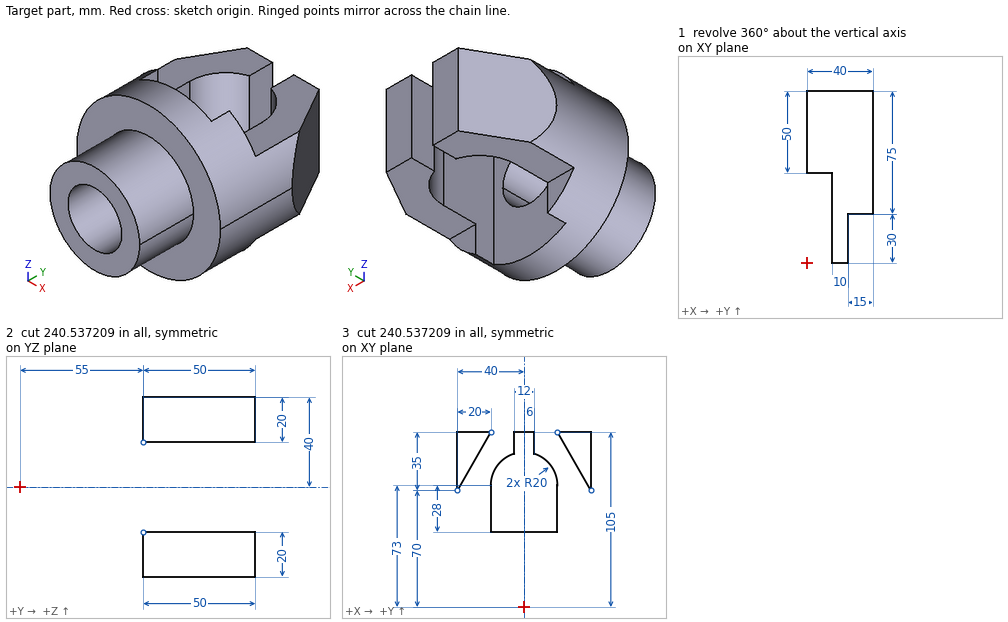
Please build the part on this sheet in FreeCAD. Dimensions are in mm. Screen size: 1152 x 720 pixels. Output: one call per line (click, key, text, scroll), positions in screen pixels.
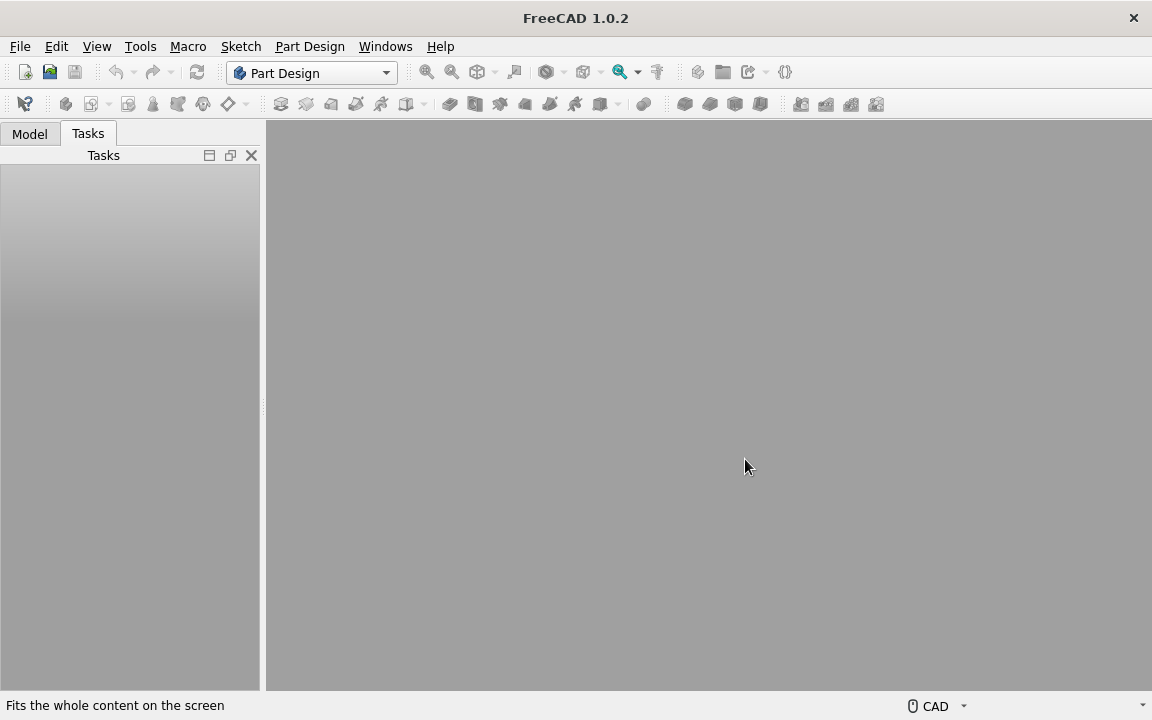
click(25, 72)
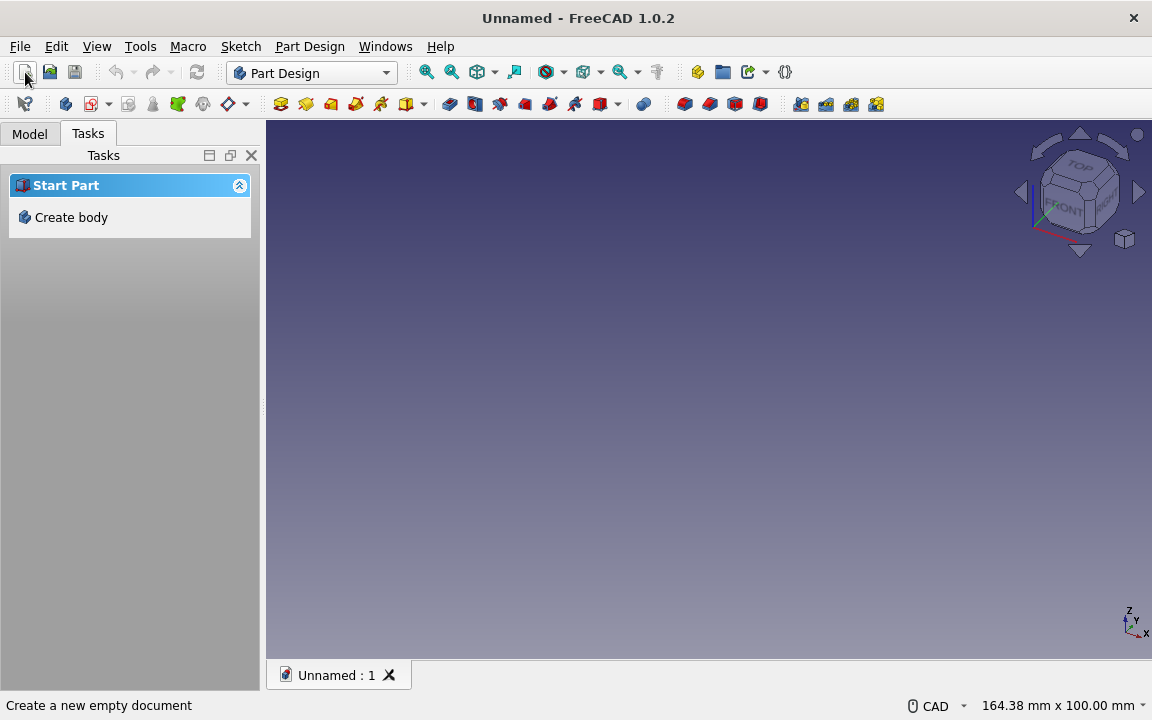
click(90, 104)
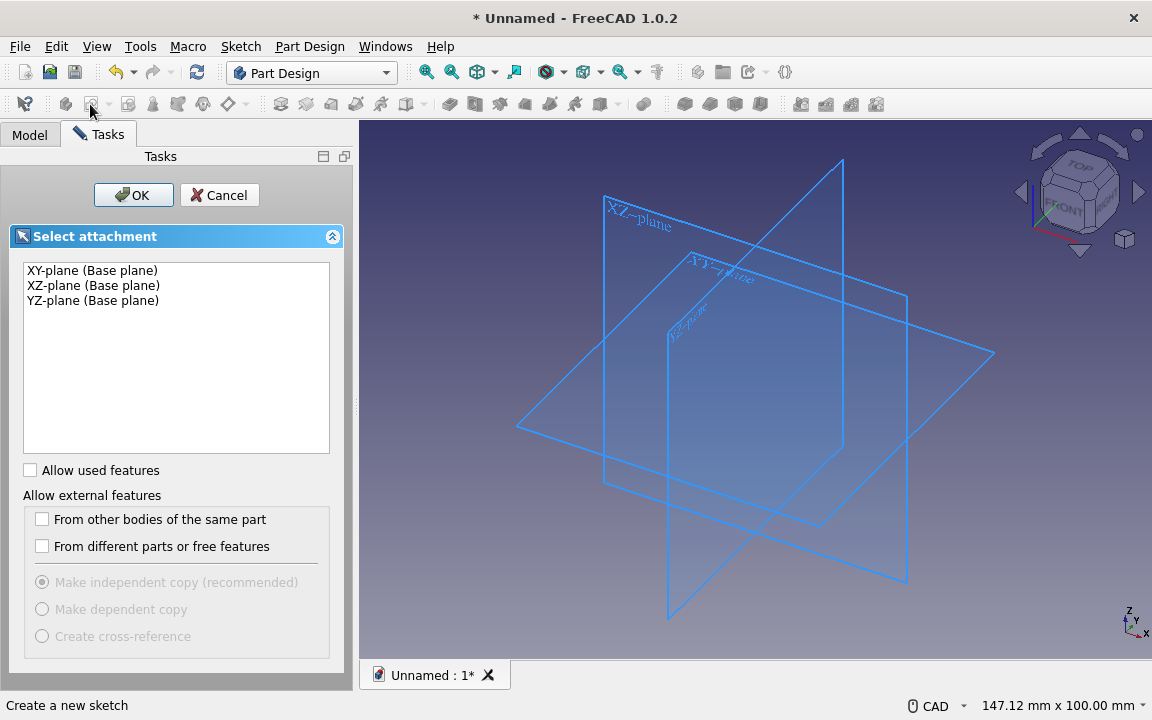
click(84, 270)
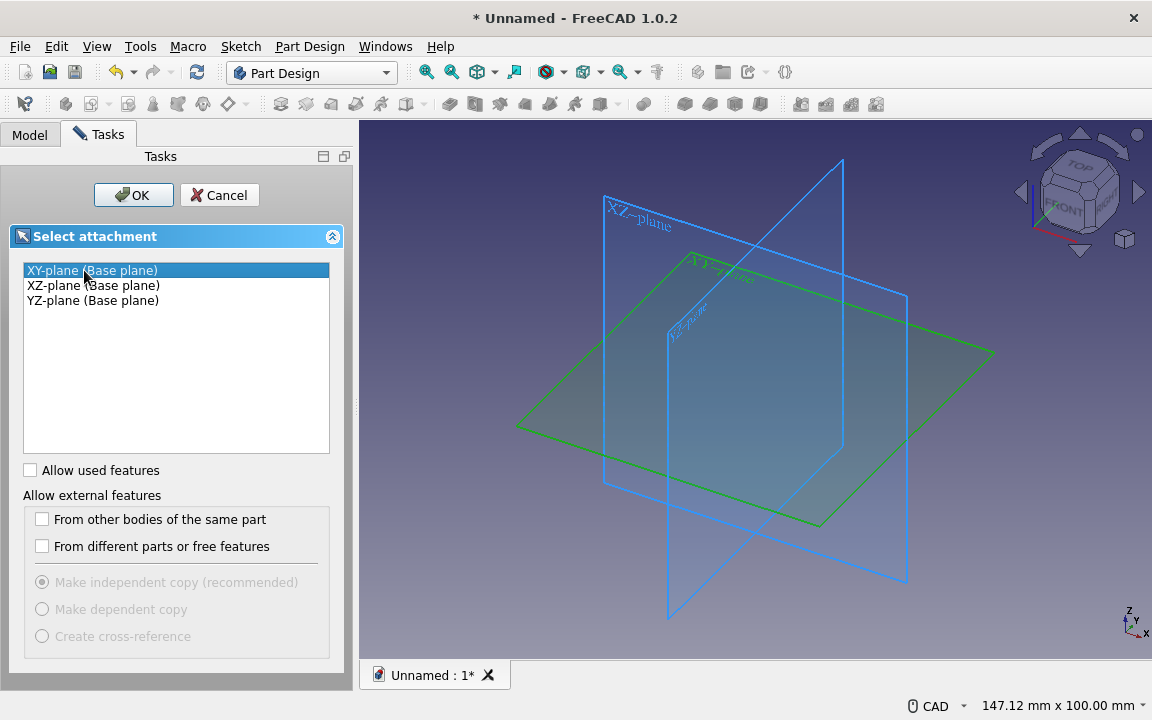
click(134, 195)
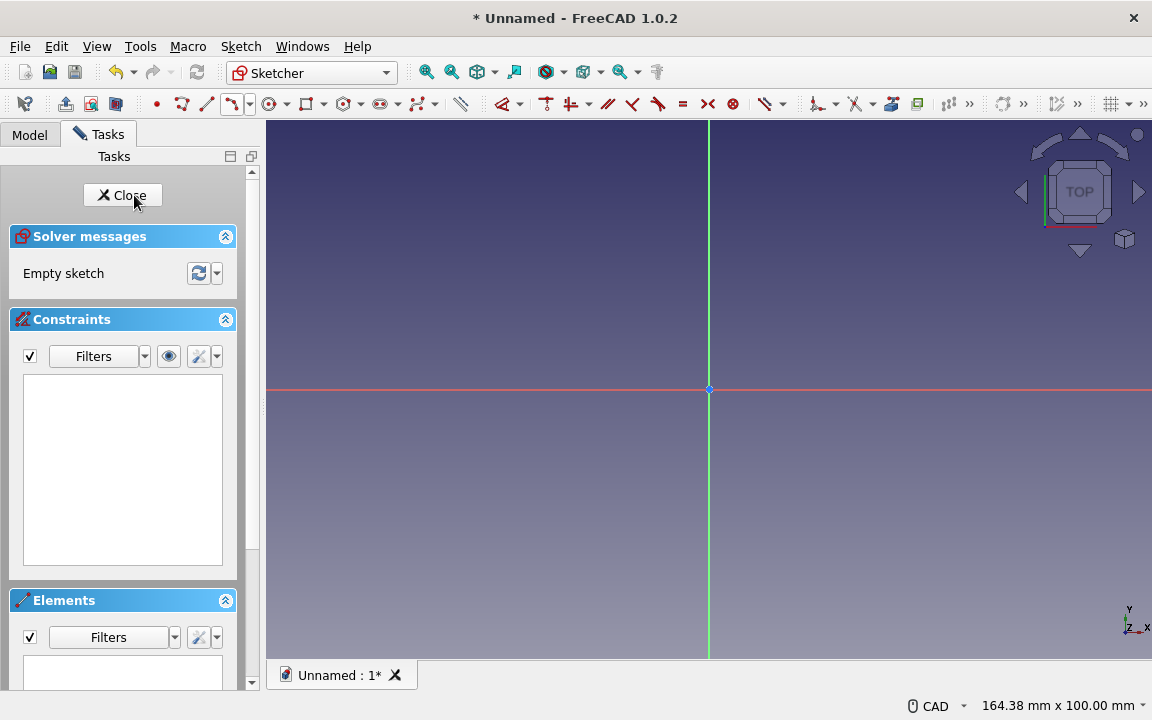
scroll(426, 631, down, 3)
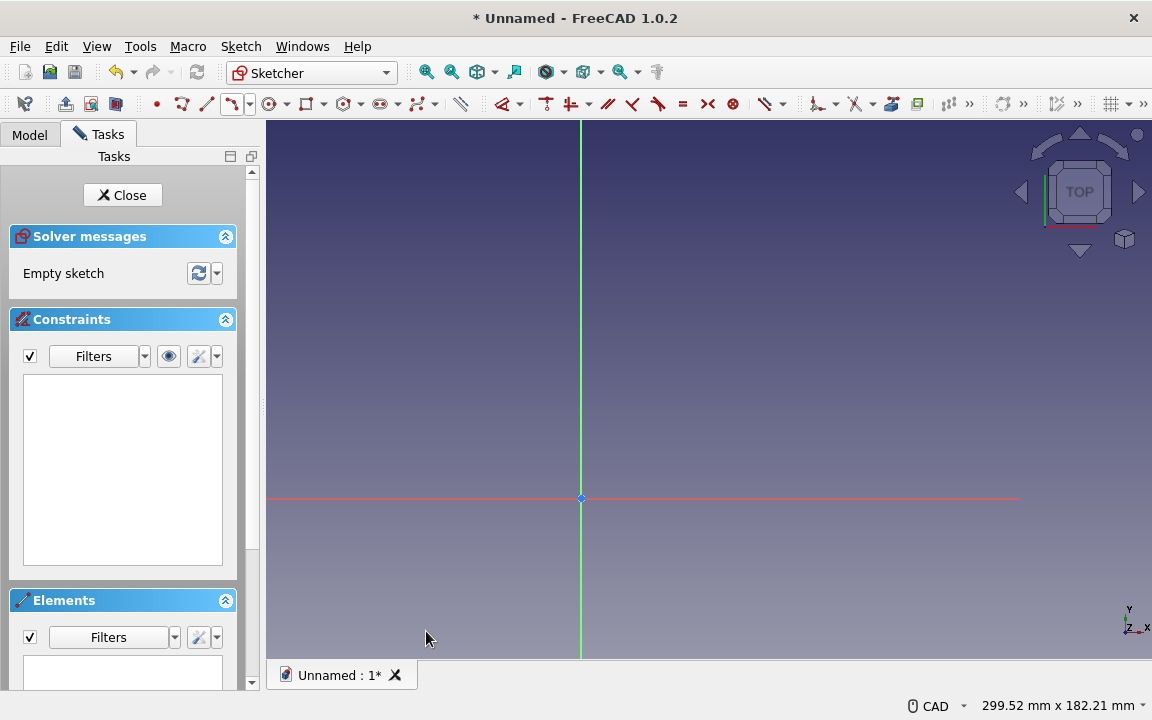
click(182, 104)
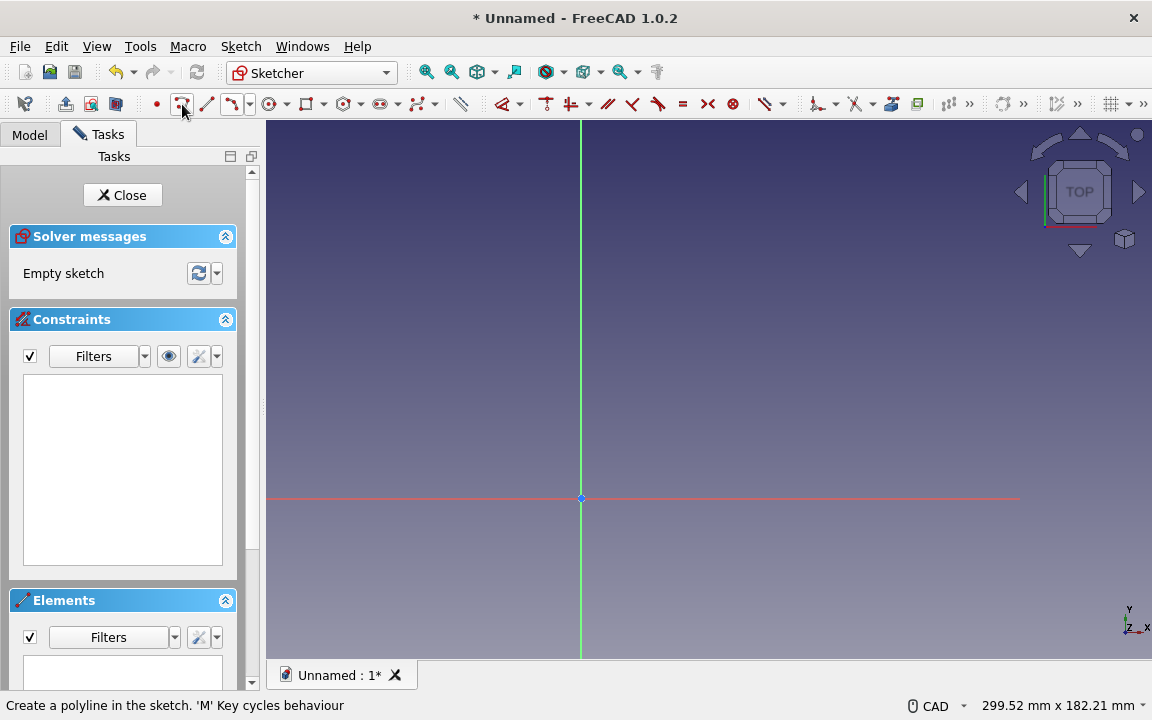
click(626, 499)
click(655, 490)
click(655, 410)
click(700, 410)
click(700, 188)
click(581, 188)
click(590, 336)
click(626, 336)
click(626, 499)
key(Escape)
key(Escape)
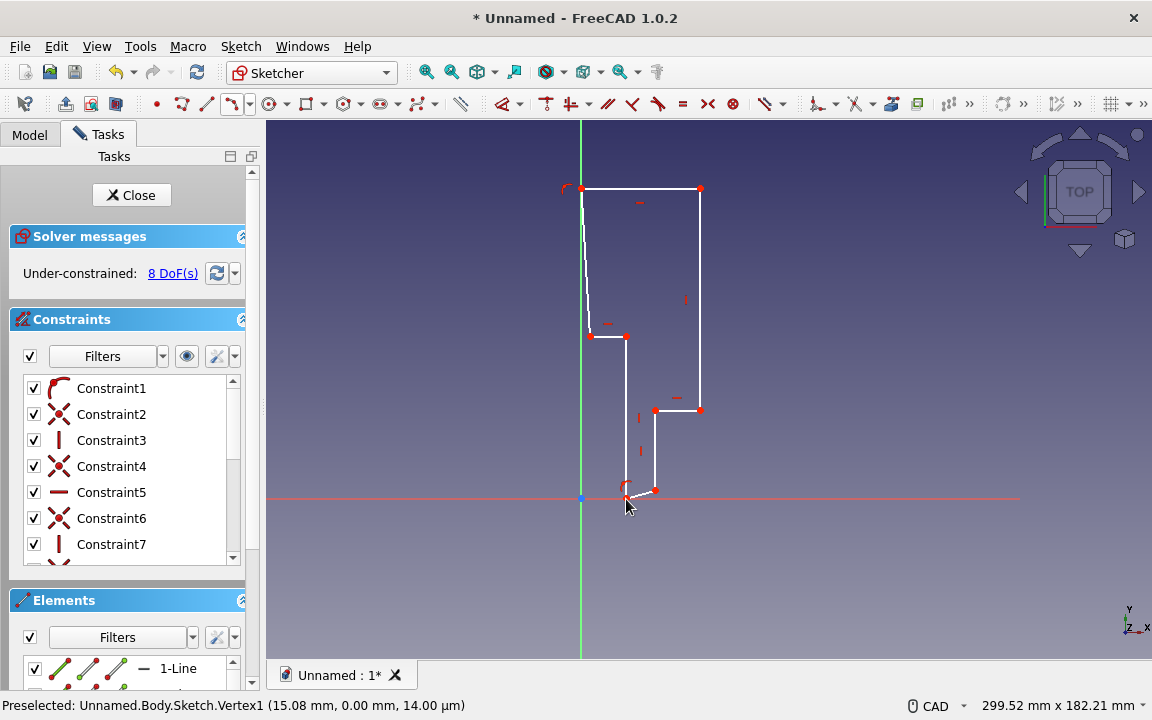
click(638, 496)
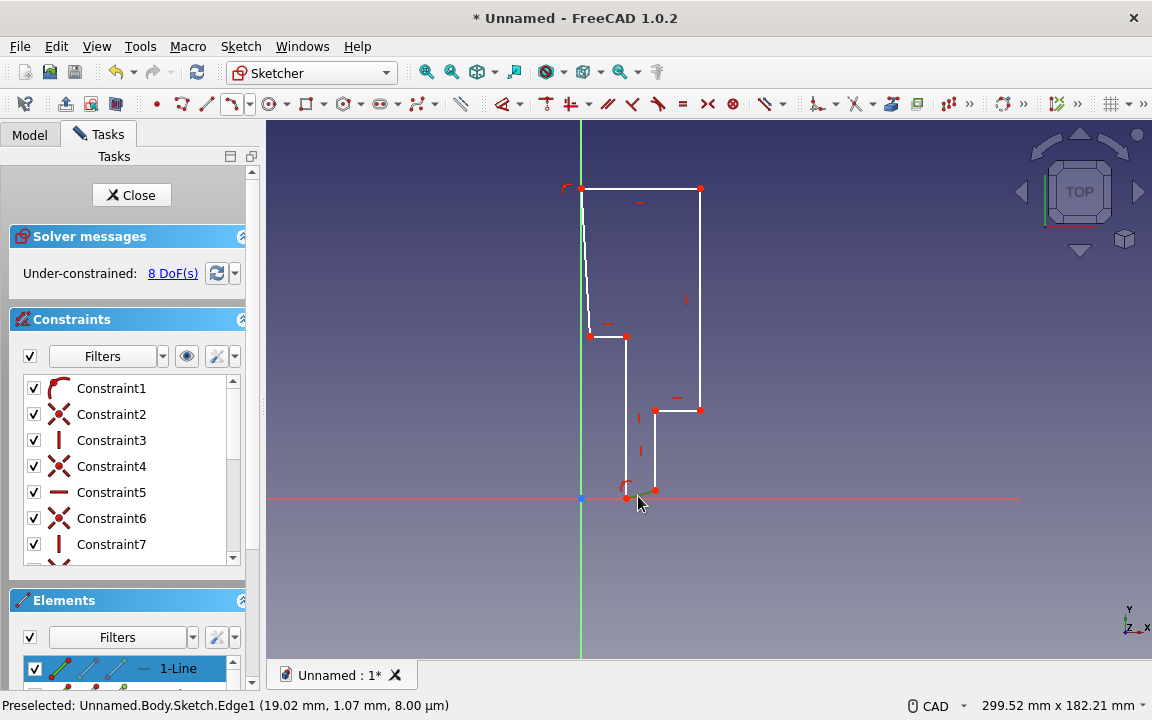
key(h)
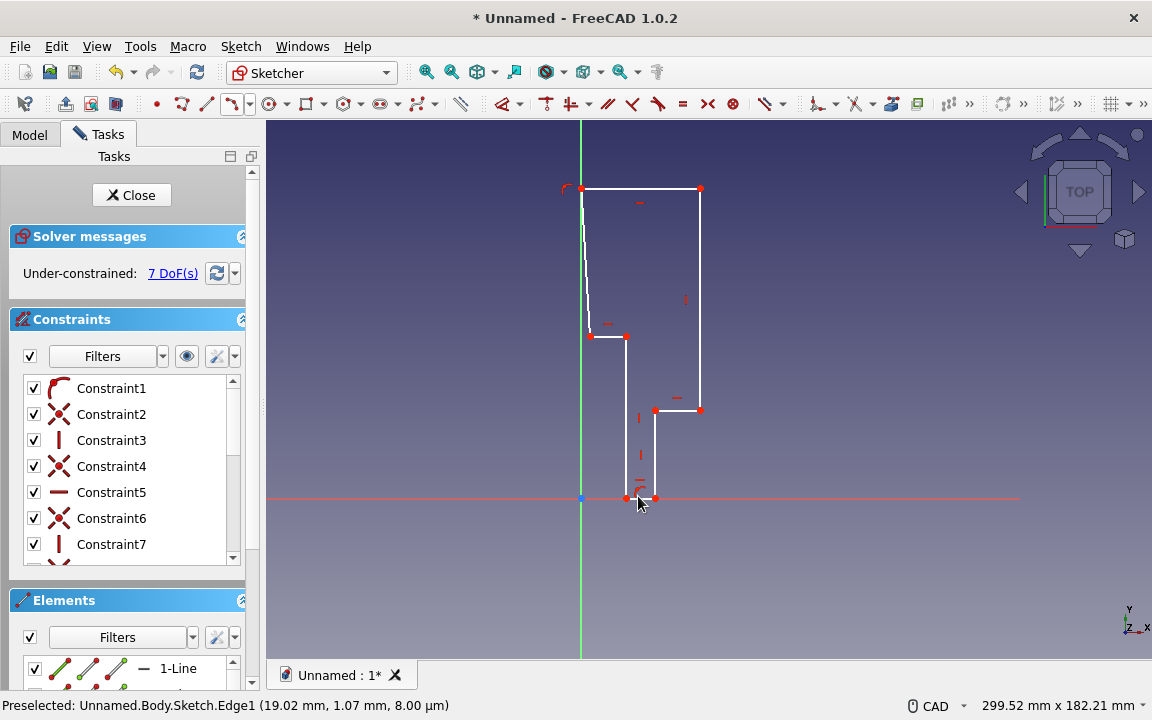
click(584, 233)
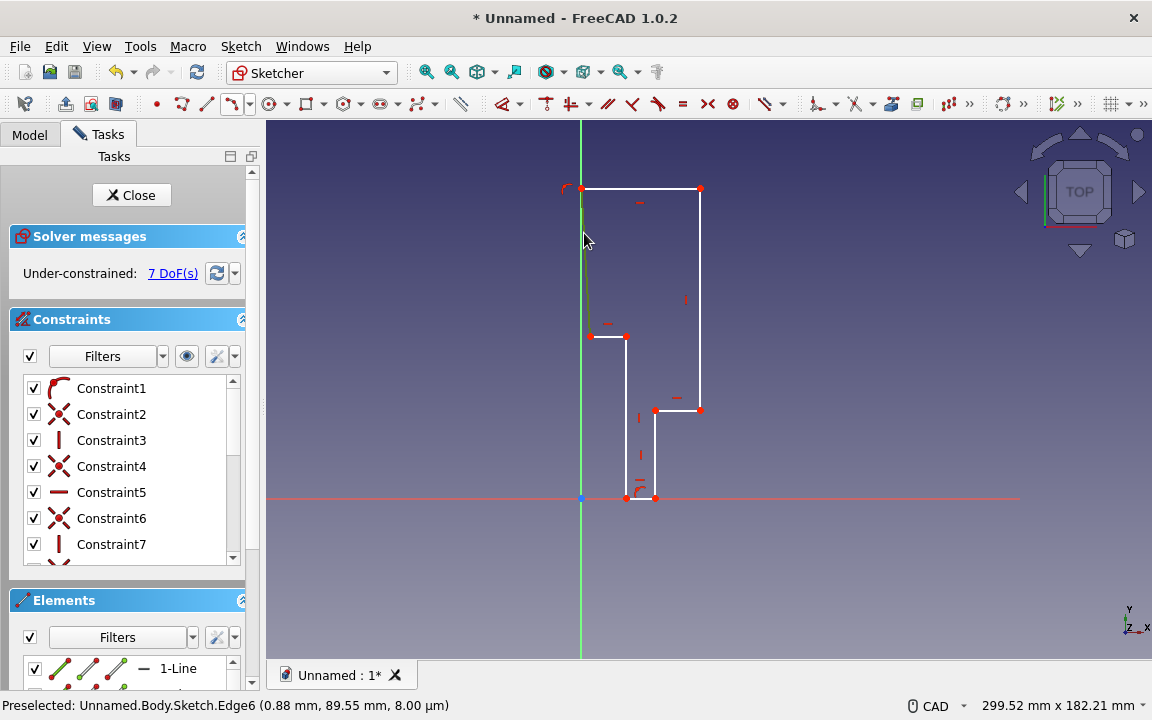
click(588, 104)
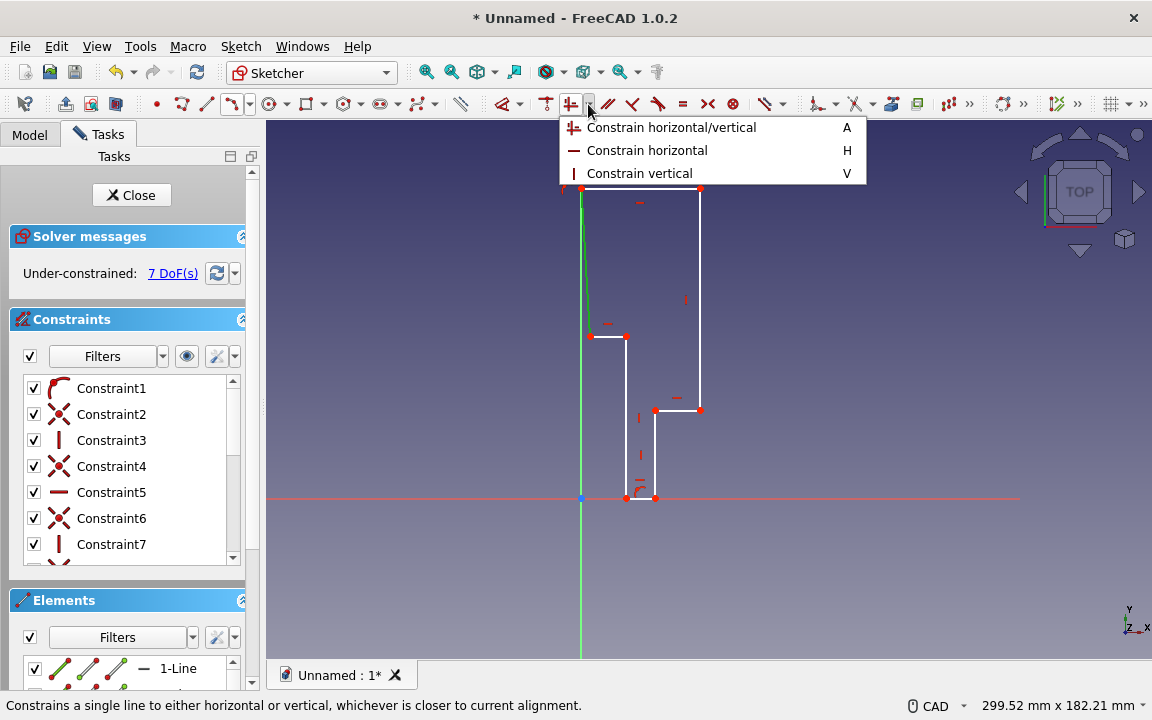
click(713, 174)